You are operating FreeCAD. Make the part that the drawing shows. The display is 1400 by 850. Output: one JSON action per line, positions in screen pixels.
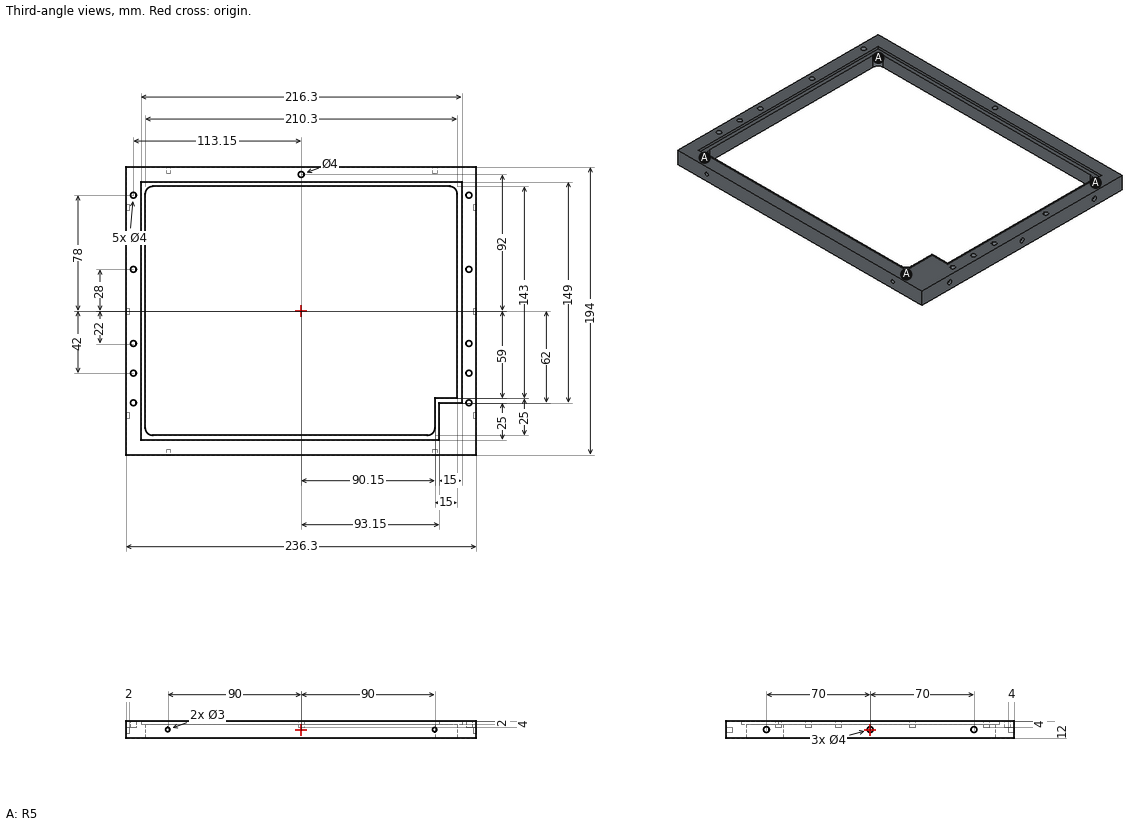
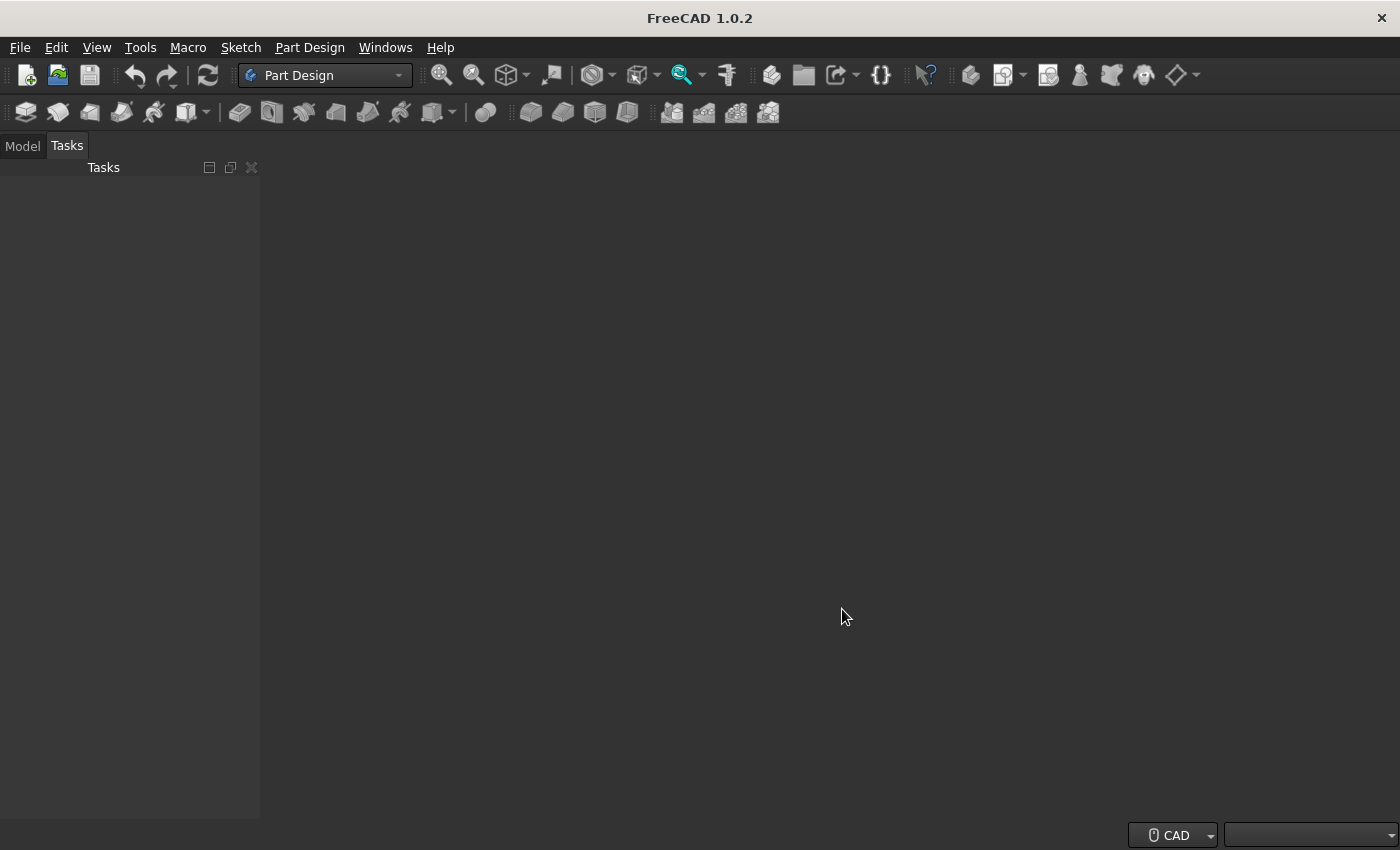
{"action": "left_click", "coordinate": [26, 76]}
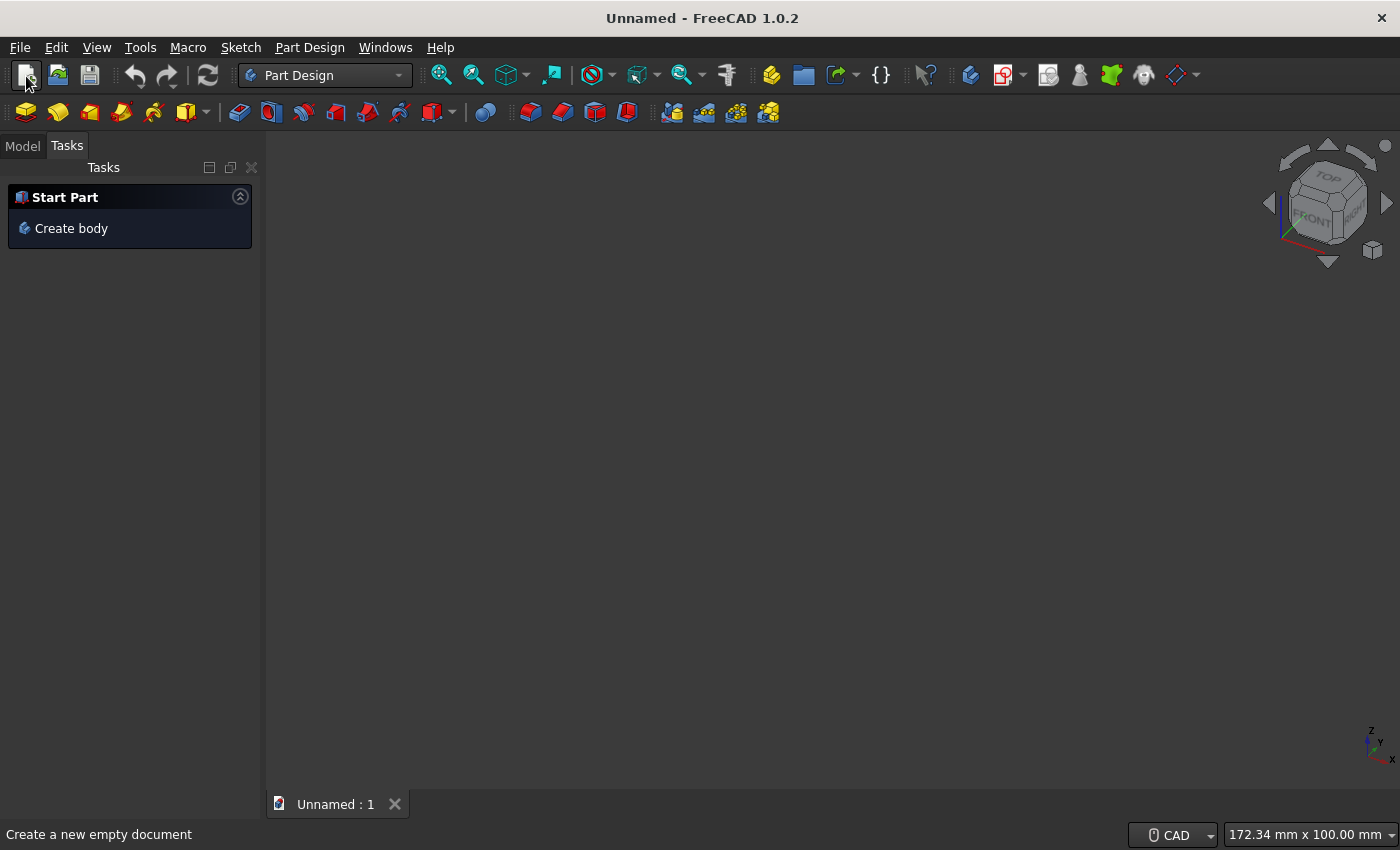
{"action": "left_click", "coordinate": [1004, 76]}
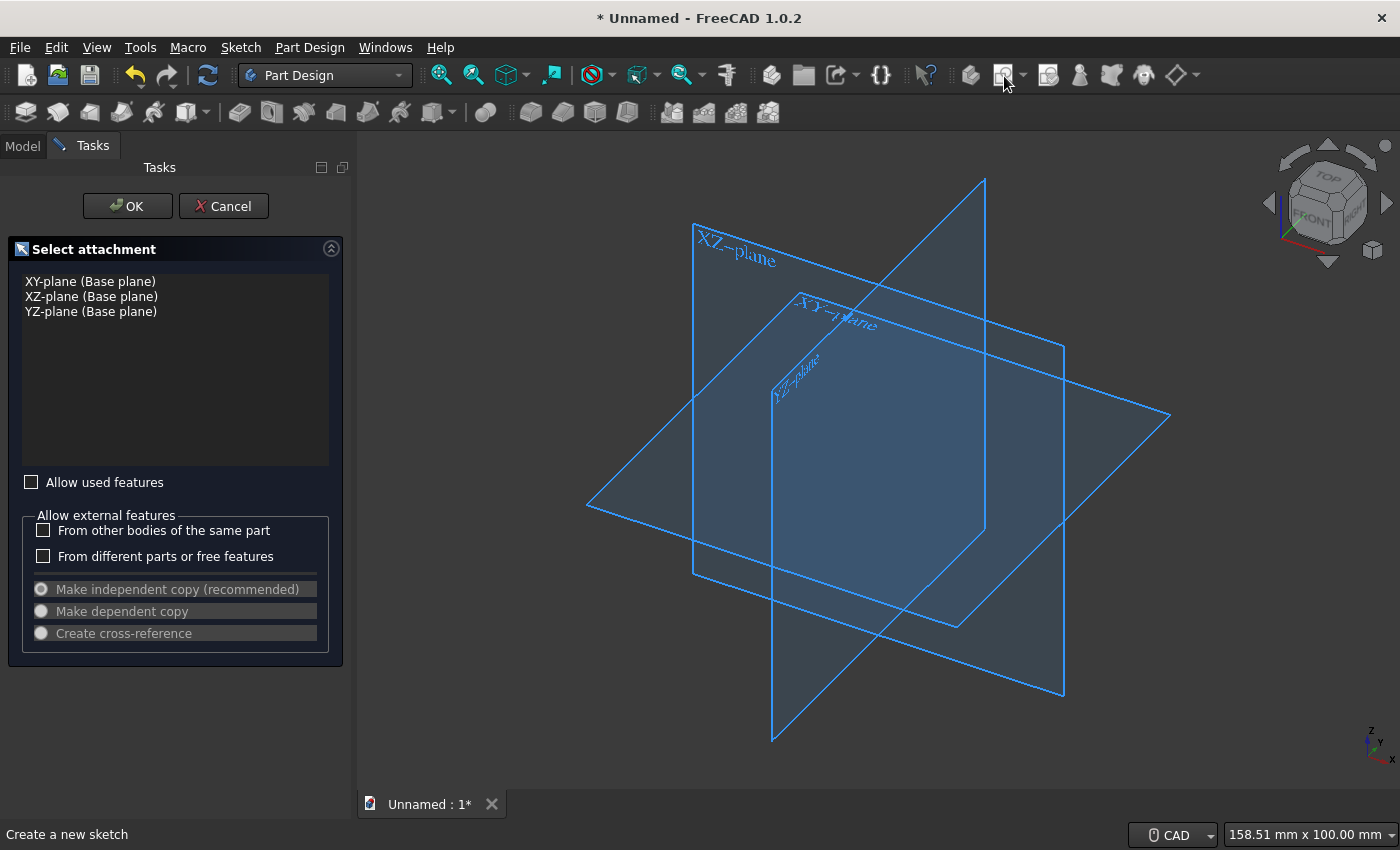
{"action": "left_click", "coordinate": [82, 282]}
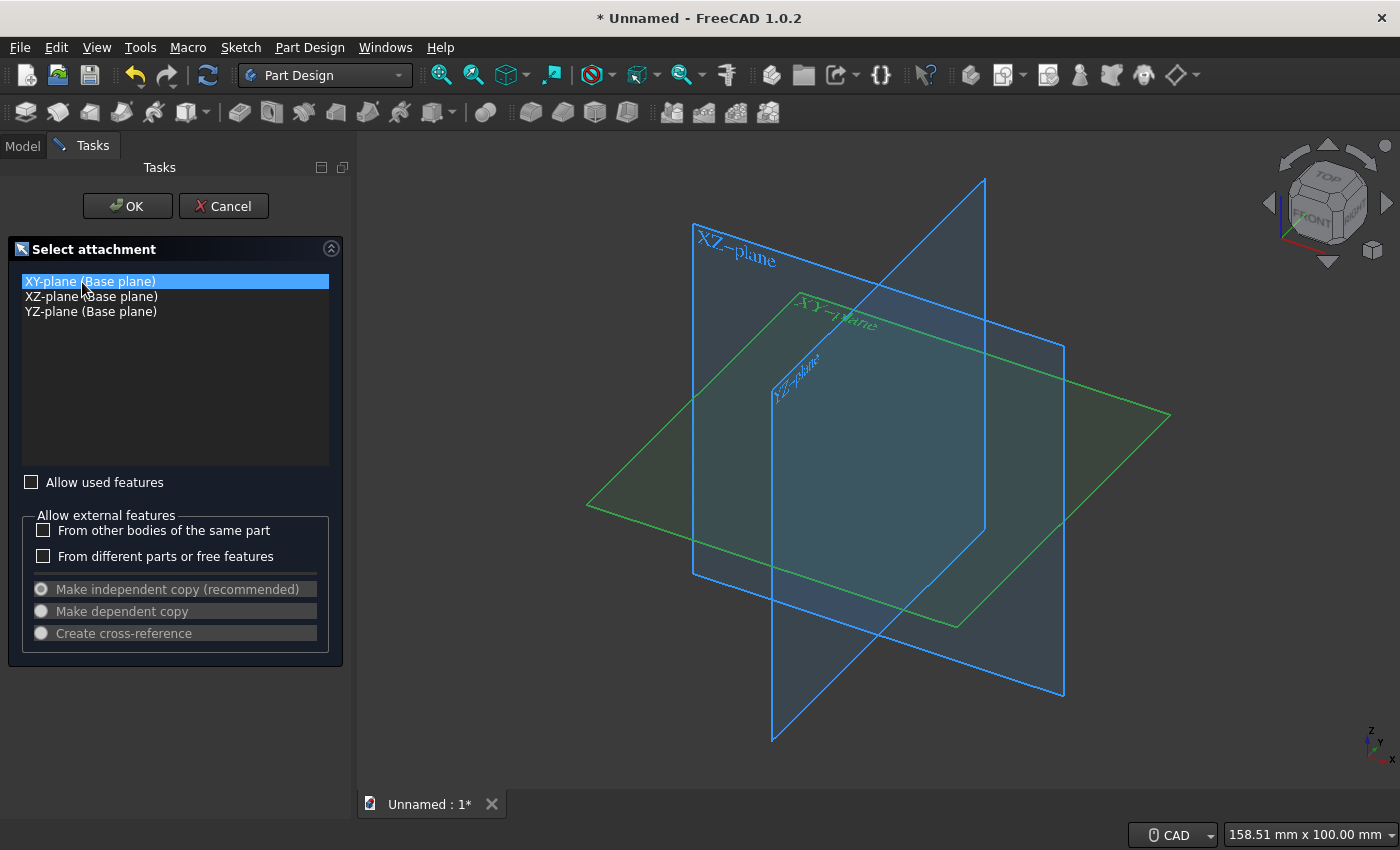
{"action": "left_click", "coordinate": [128, 206]}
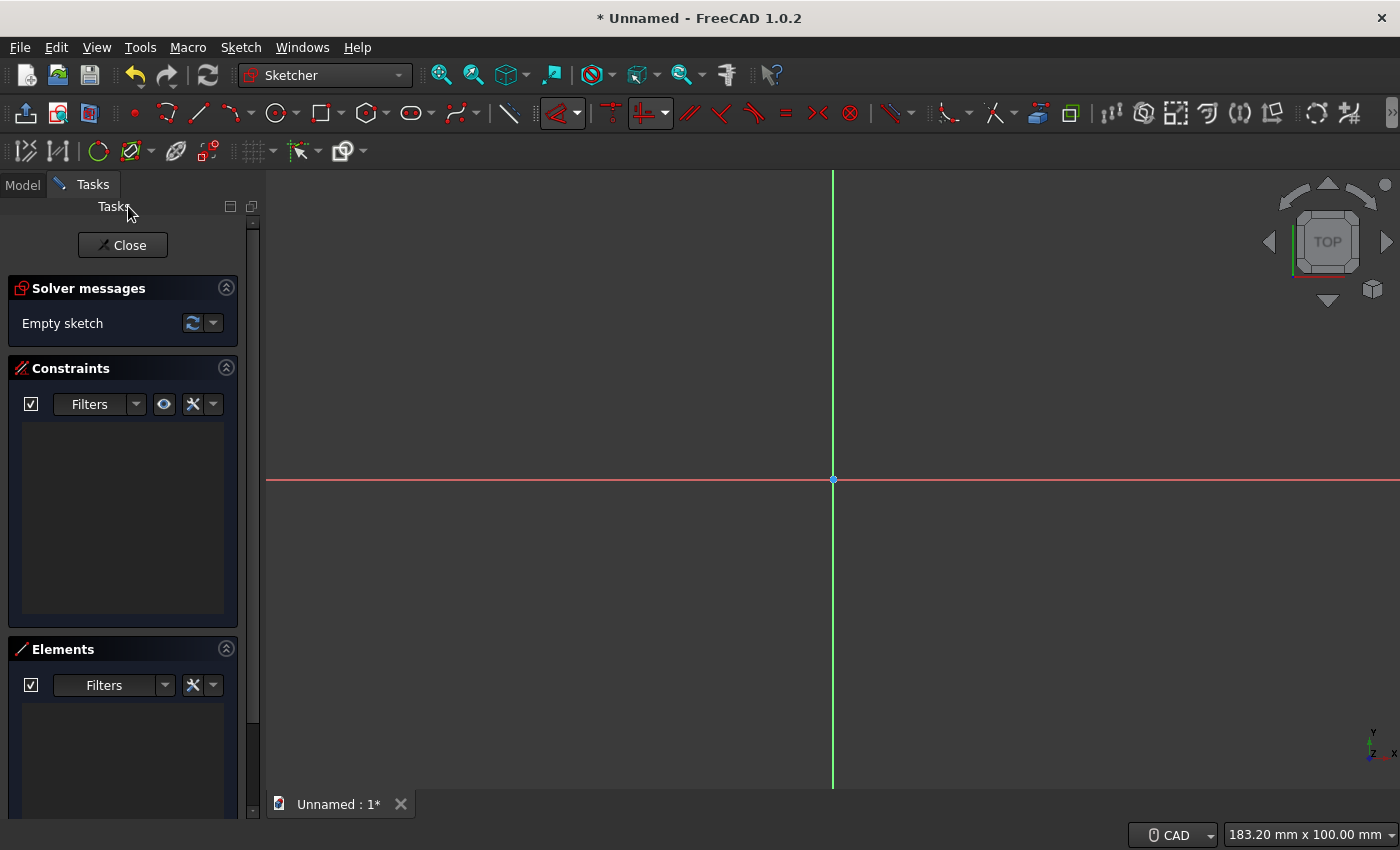
{"action": "scroll", "coordinate": [735, 480], "scroll_direction": "down", "scroll_amount": 6}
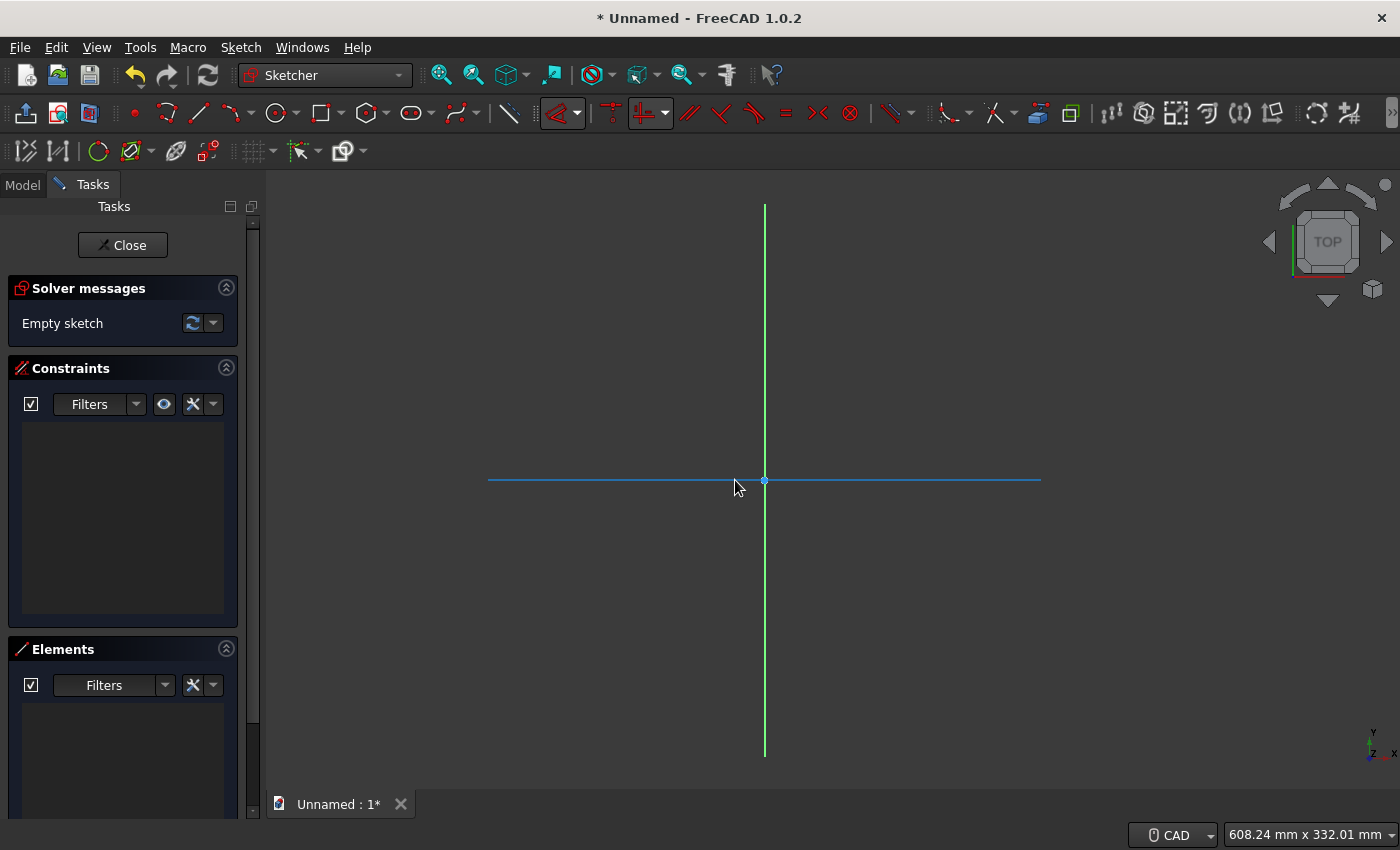
{"action": "key", "text": "g v"}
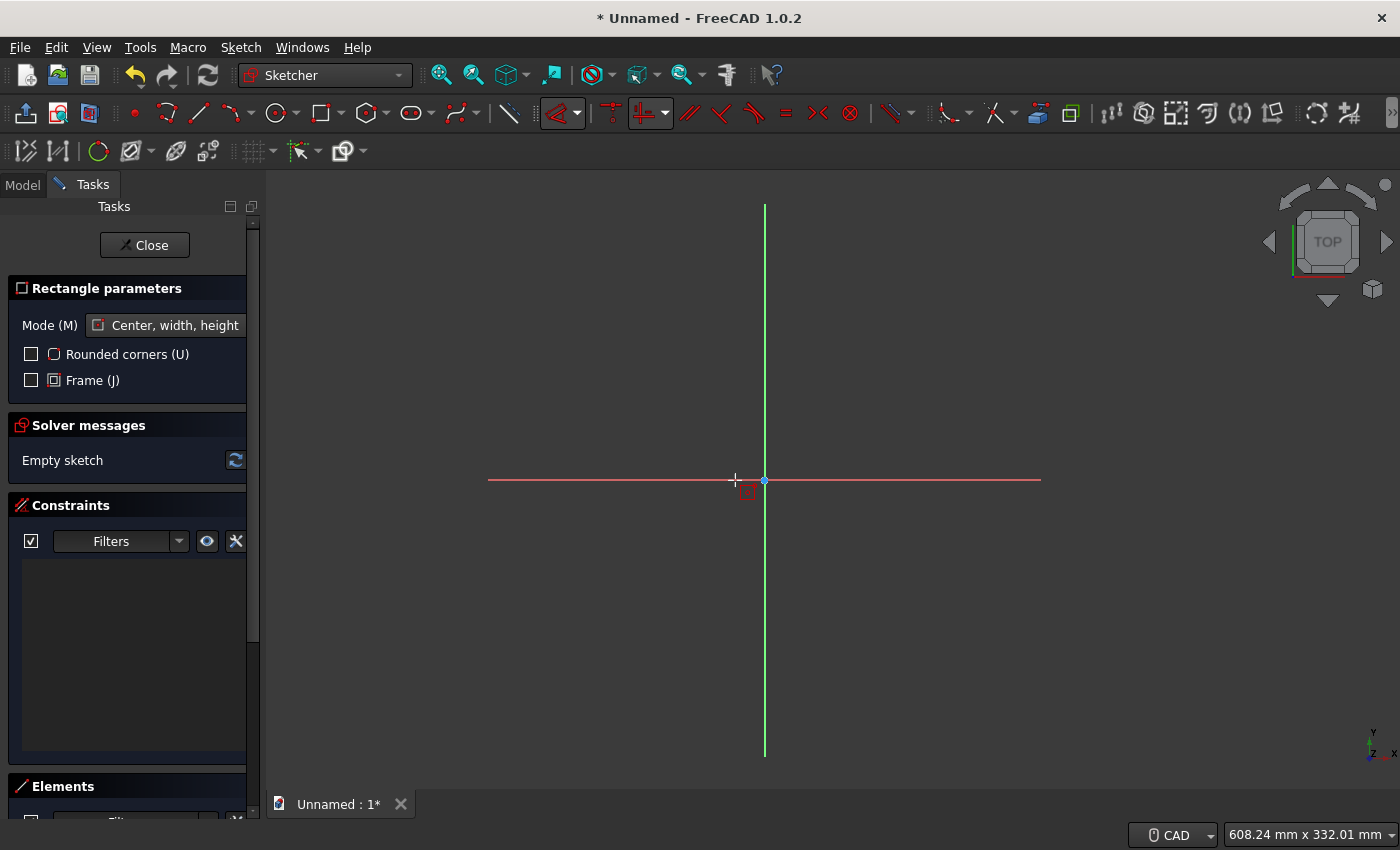
{"action": "left_click", "coordinate": [765, 480]}
{"action": "left_click", "coordinate": [985, 299]}
{"action": "key", "text": "Escape"}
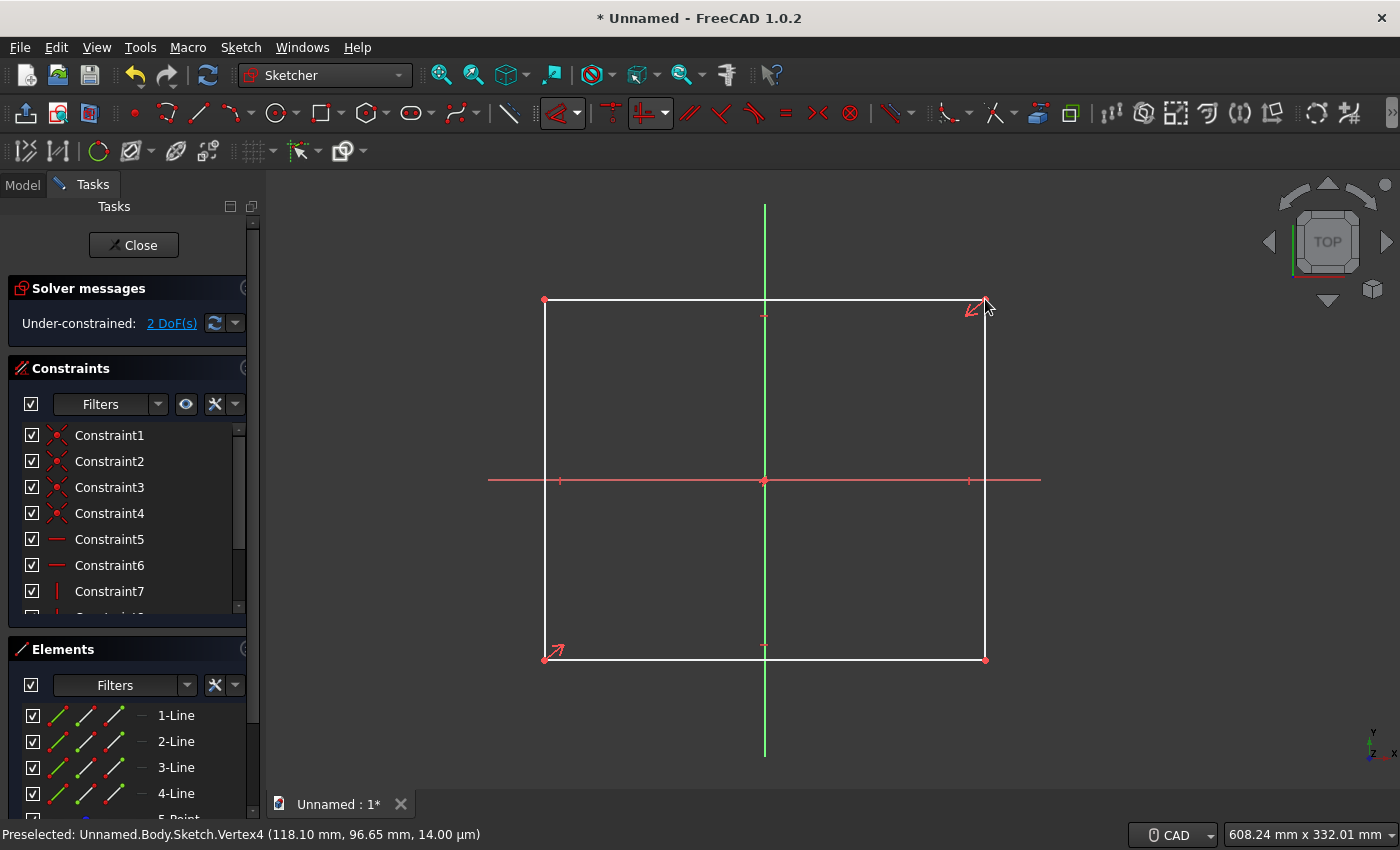
{"action": "left_click", "coordinate": [556, 114]}